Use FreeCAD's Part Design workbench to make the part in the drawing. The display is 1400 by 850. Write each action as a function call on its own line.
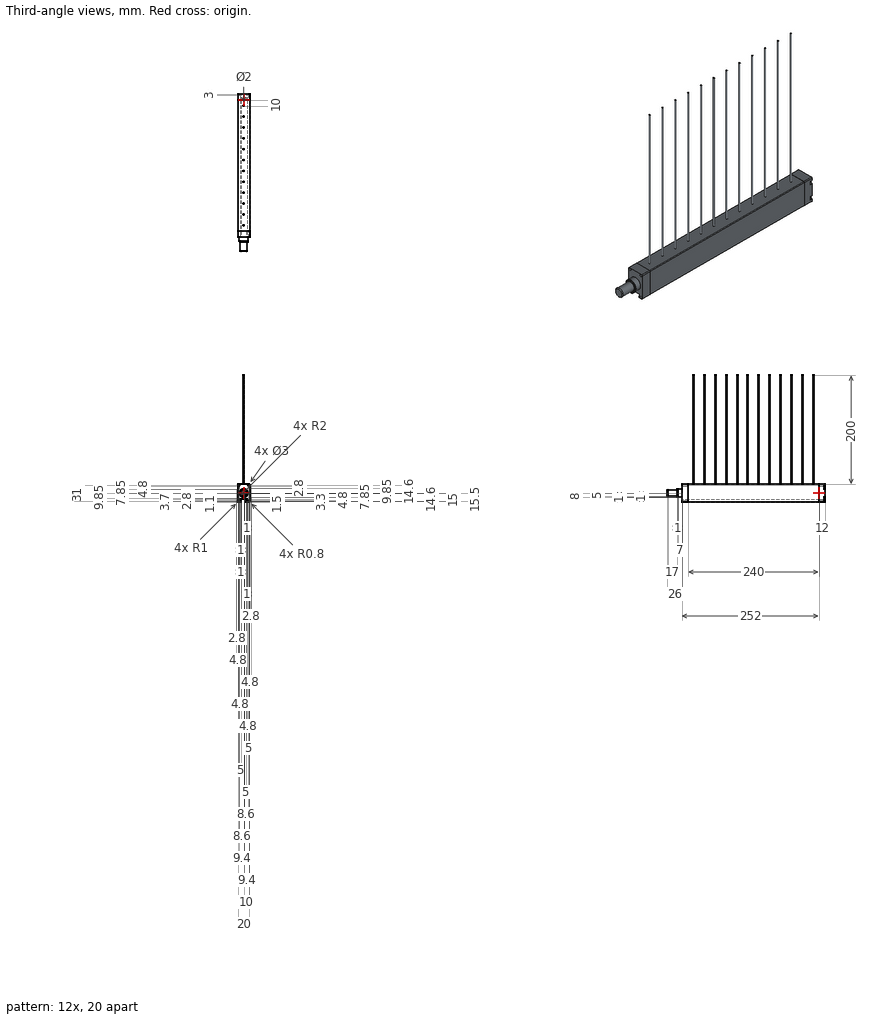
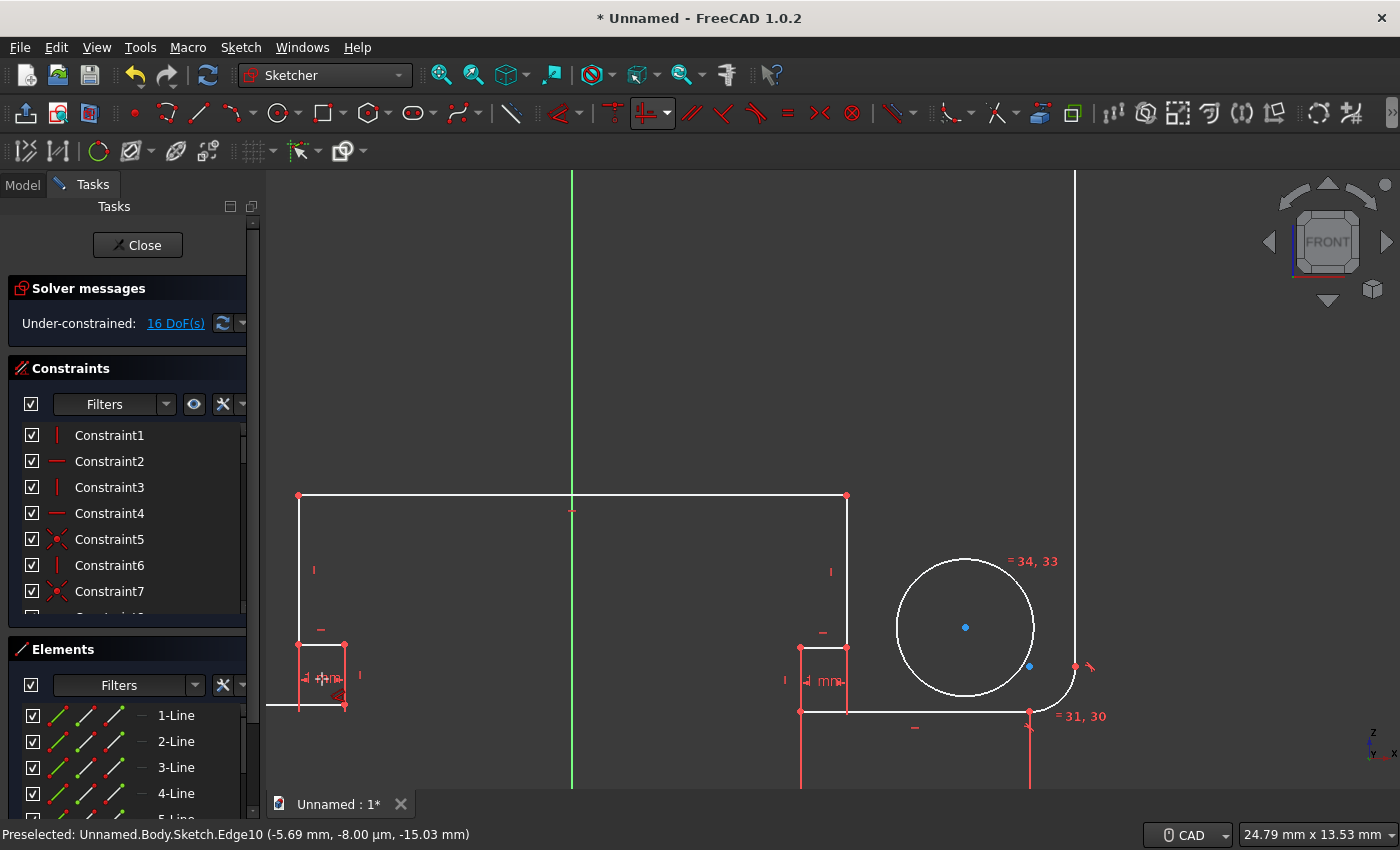
scroll(827, 651, down, 7)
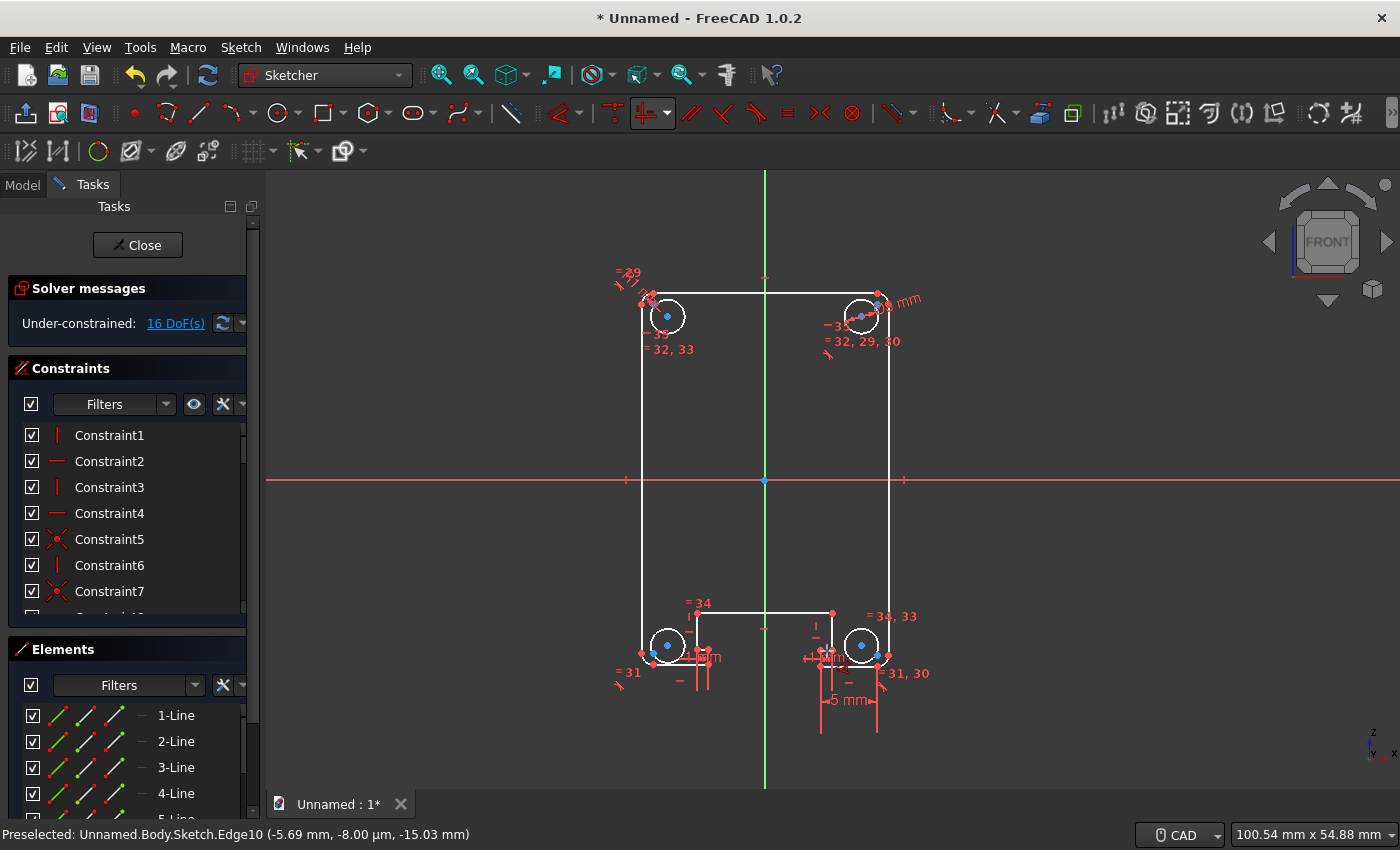
scroll(697, 665, up, 2)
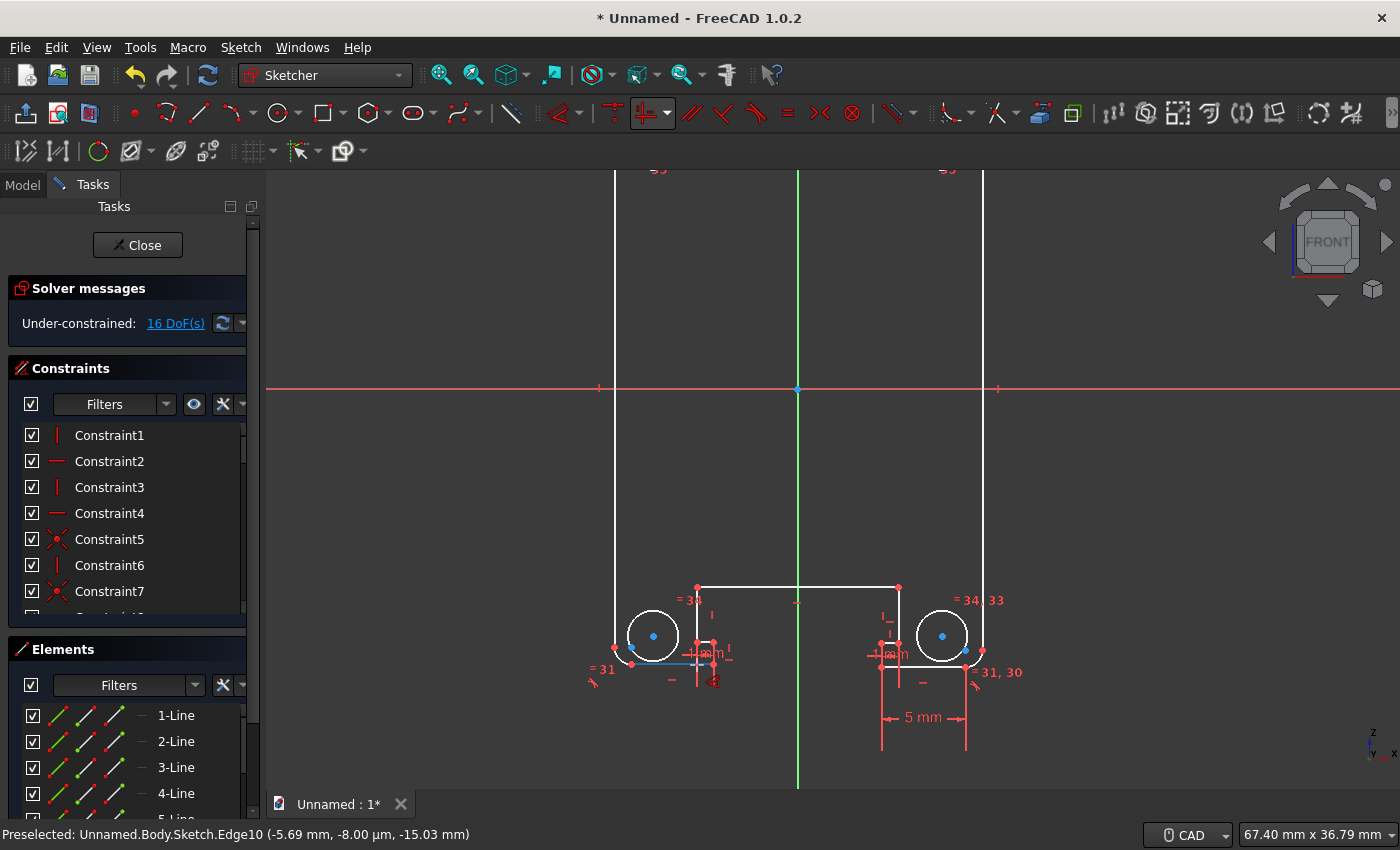
click(697, 664)
click(673, 698)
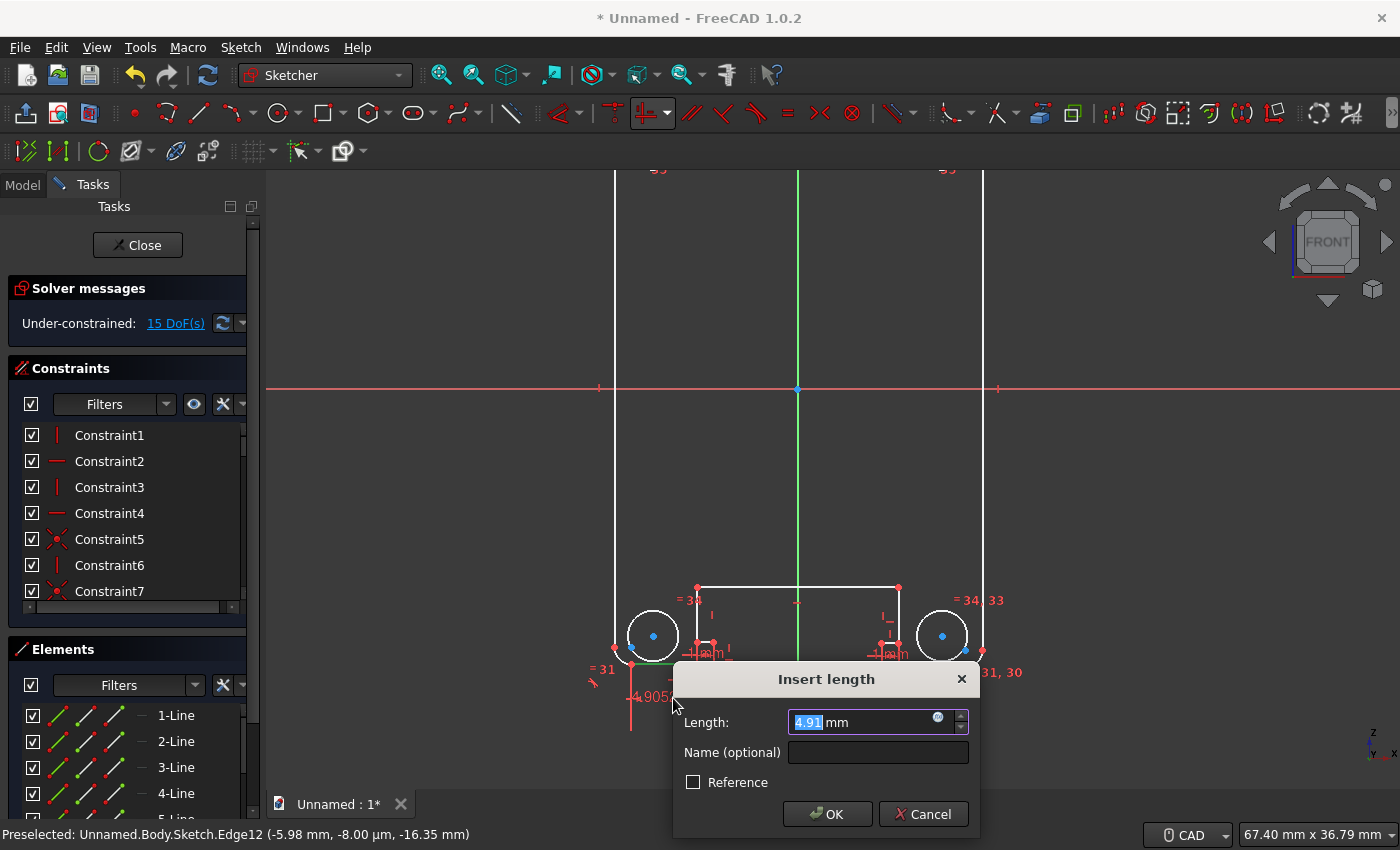
text(5)
key(Return)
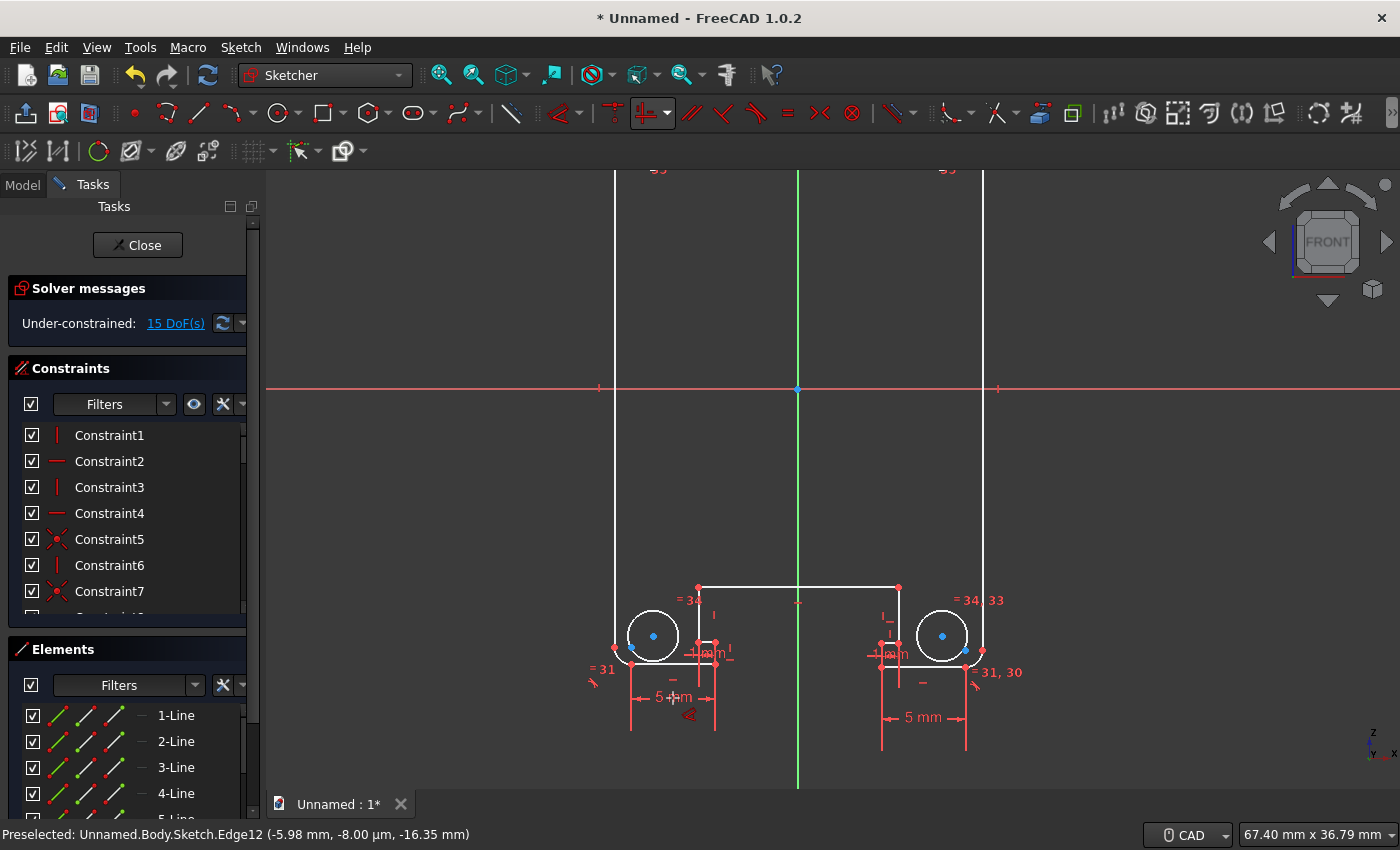
click(615, 491)
click(581, 423)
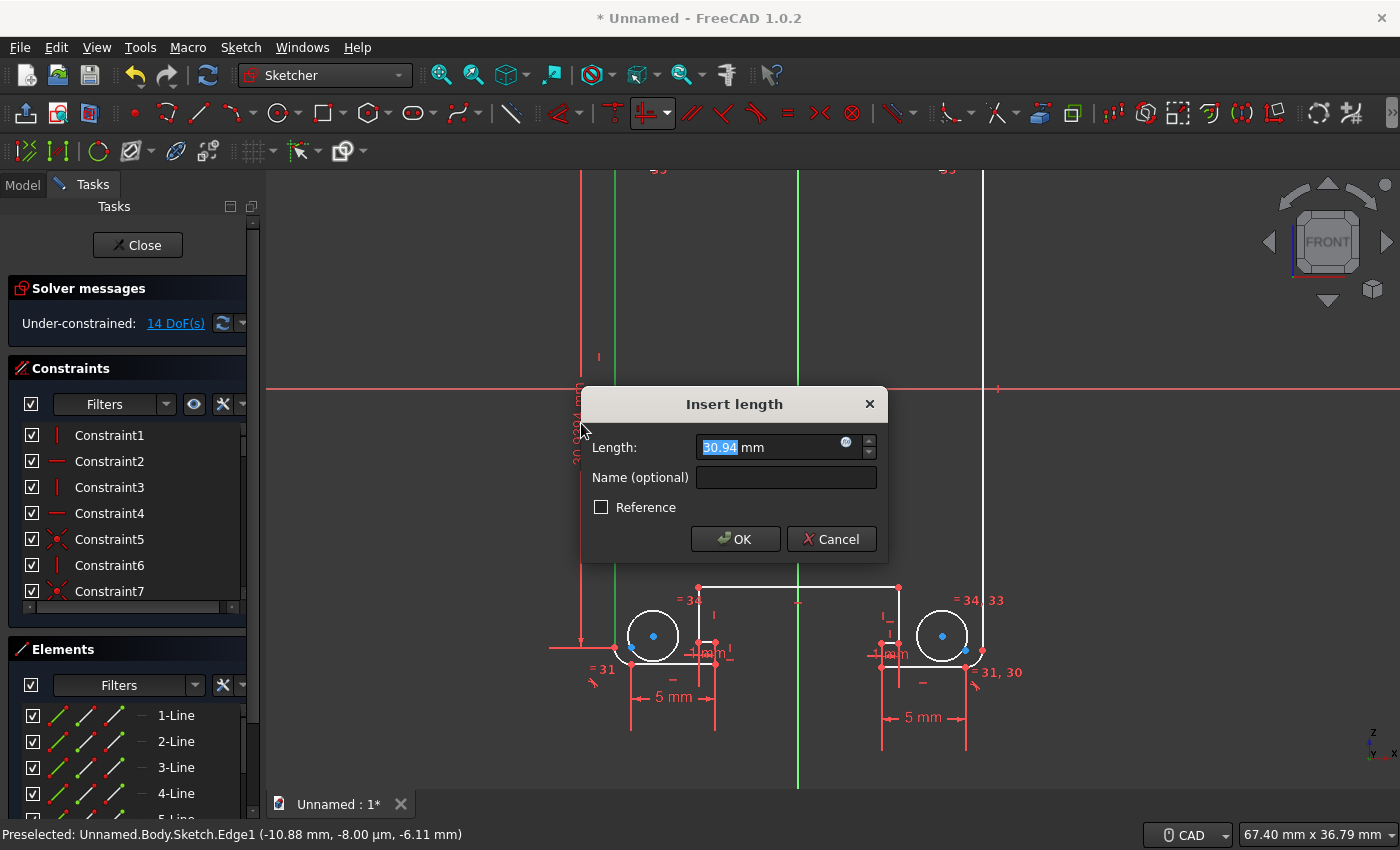
text(31)
key(Return)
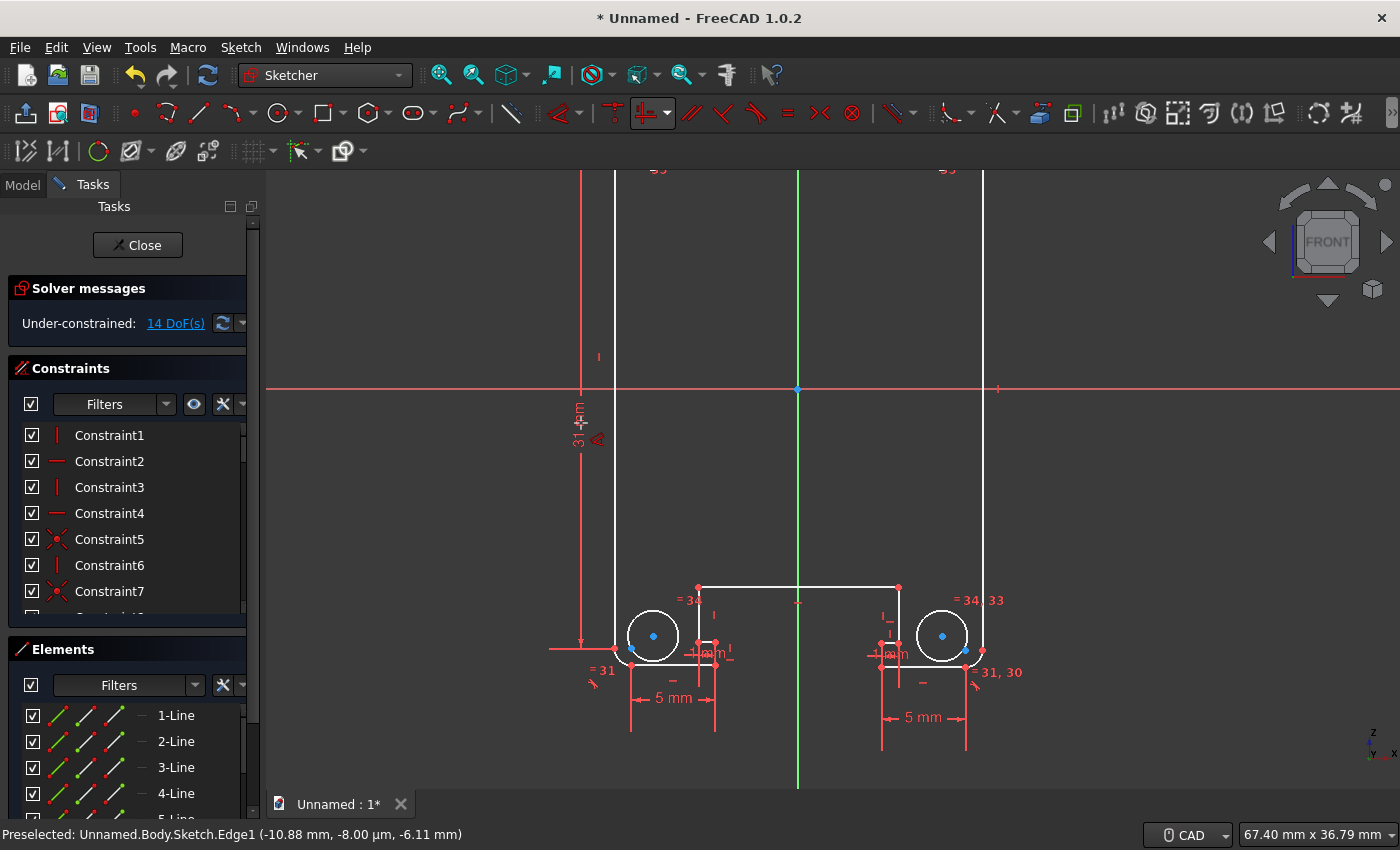
scroll(697, 663, down, 2)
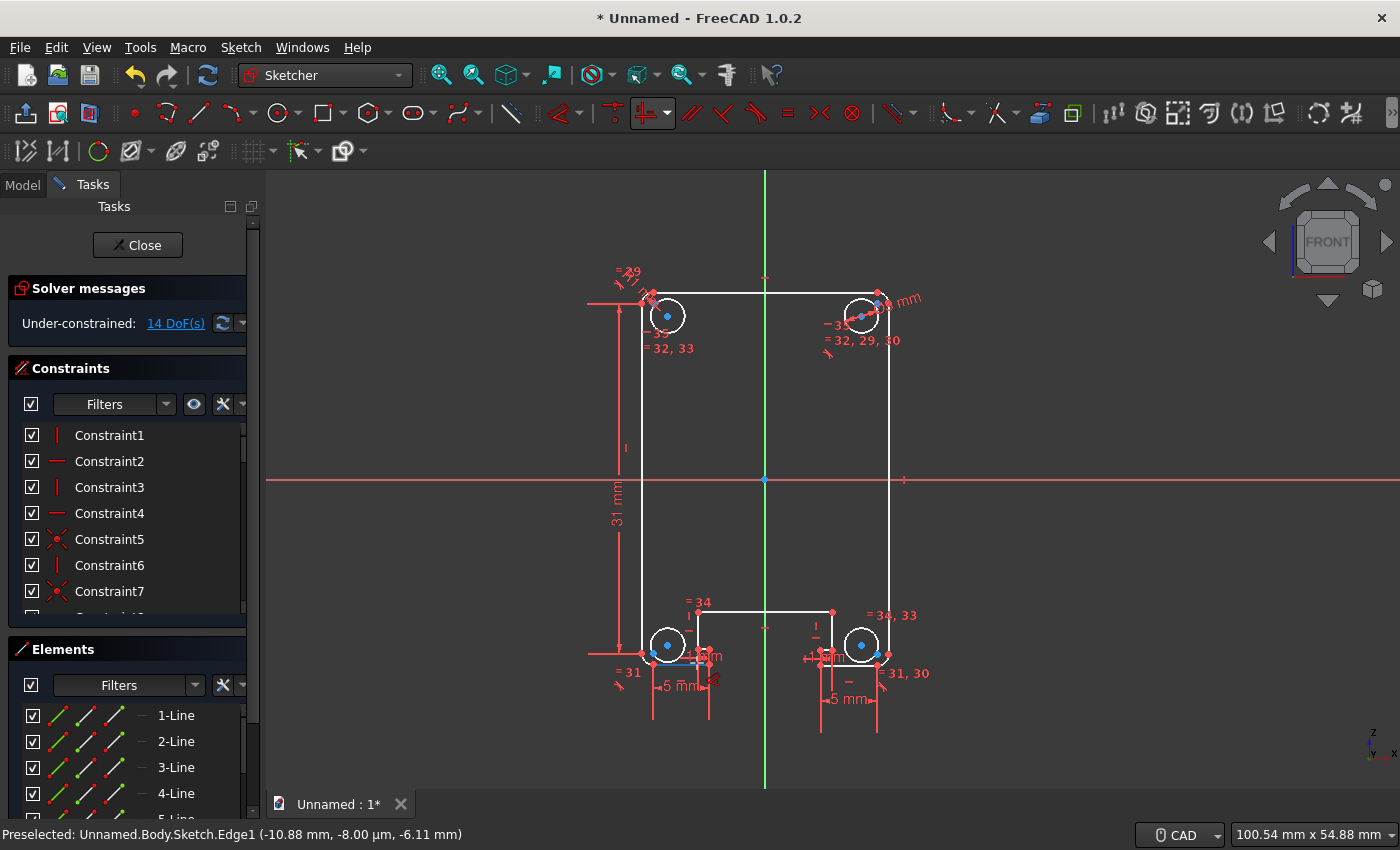
click(720, 293)
click(714, 259)